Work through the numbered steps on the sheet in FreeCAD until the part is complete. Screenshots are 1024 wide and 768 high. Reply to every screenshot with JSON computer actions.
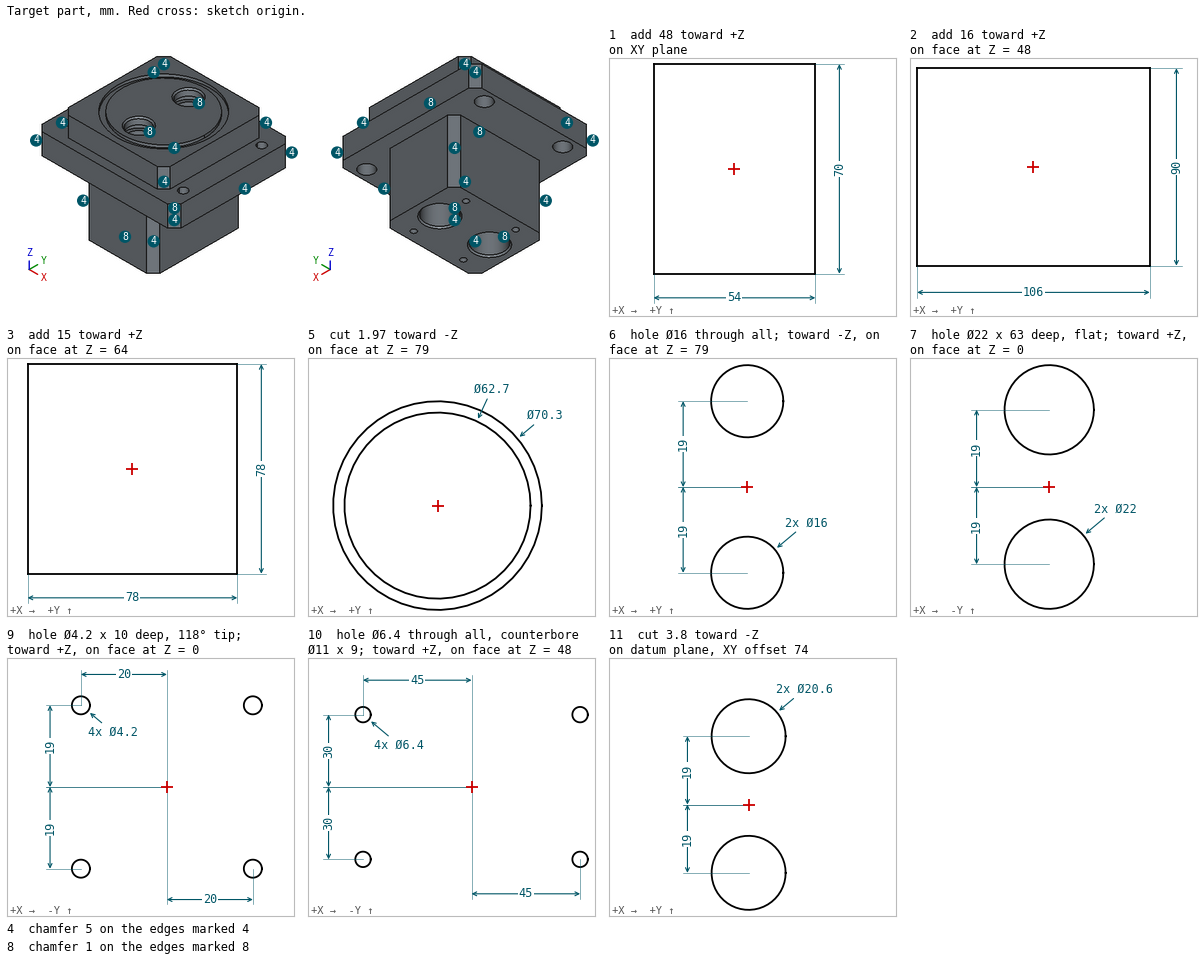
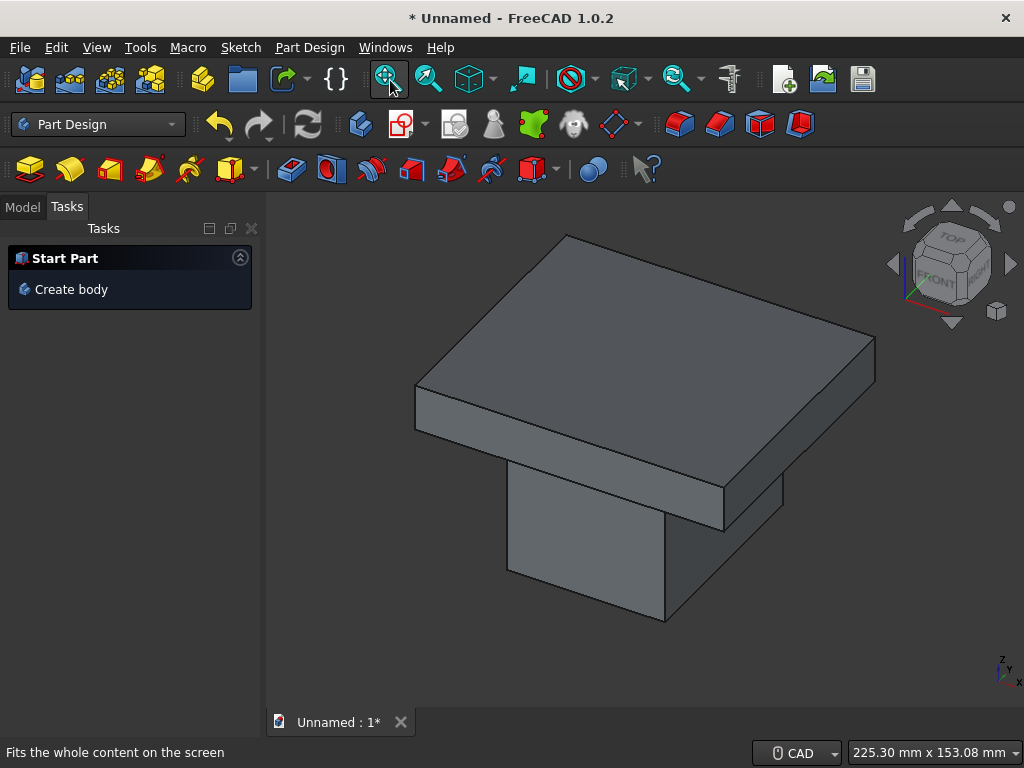
{"action": "left_click", "coordinate": [645, 360]}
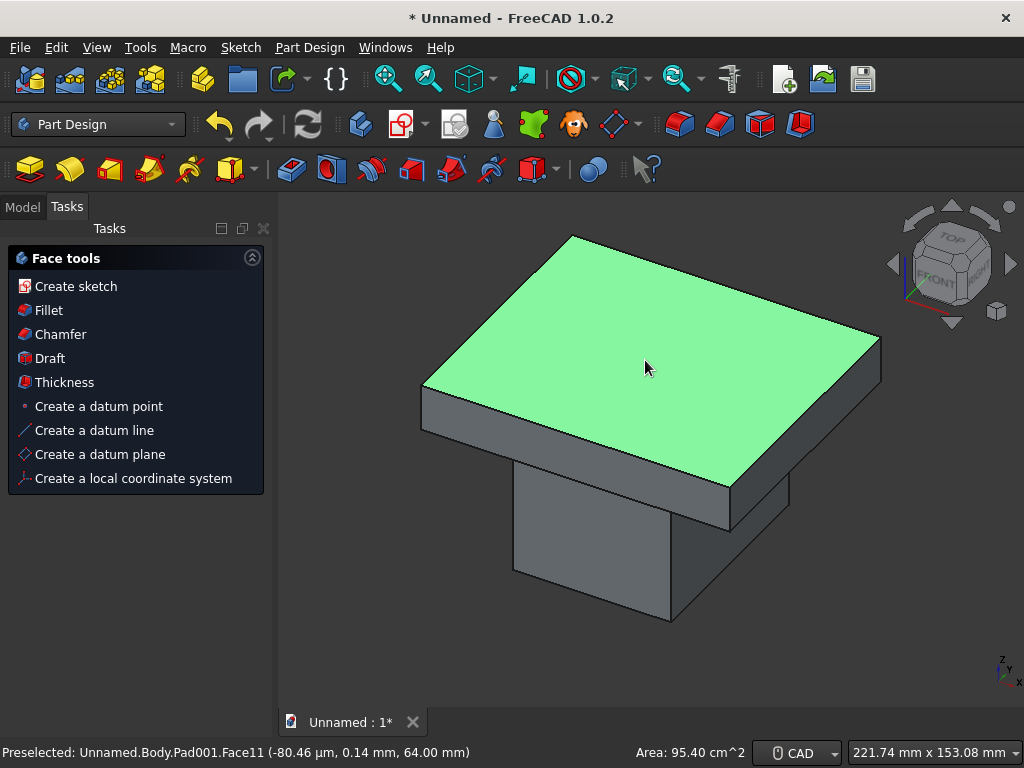
{"action": "left_click", "coordinate": [402, 124]}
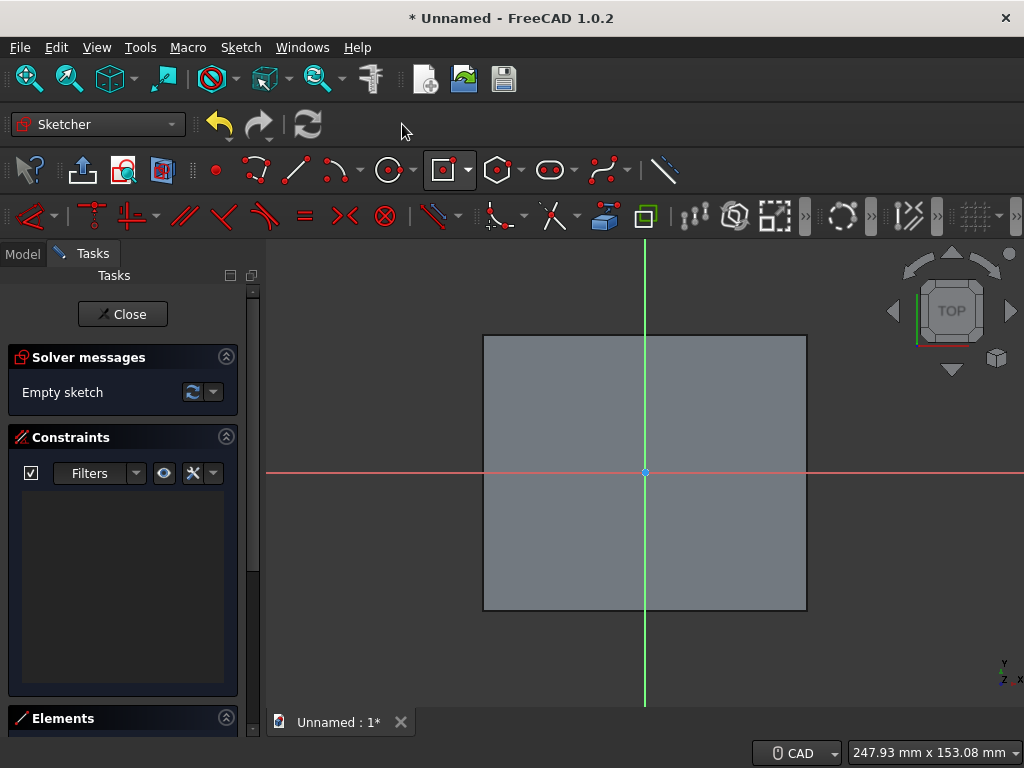
{"action": "left_click", "coordinate": [444, 170]}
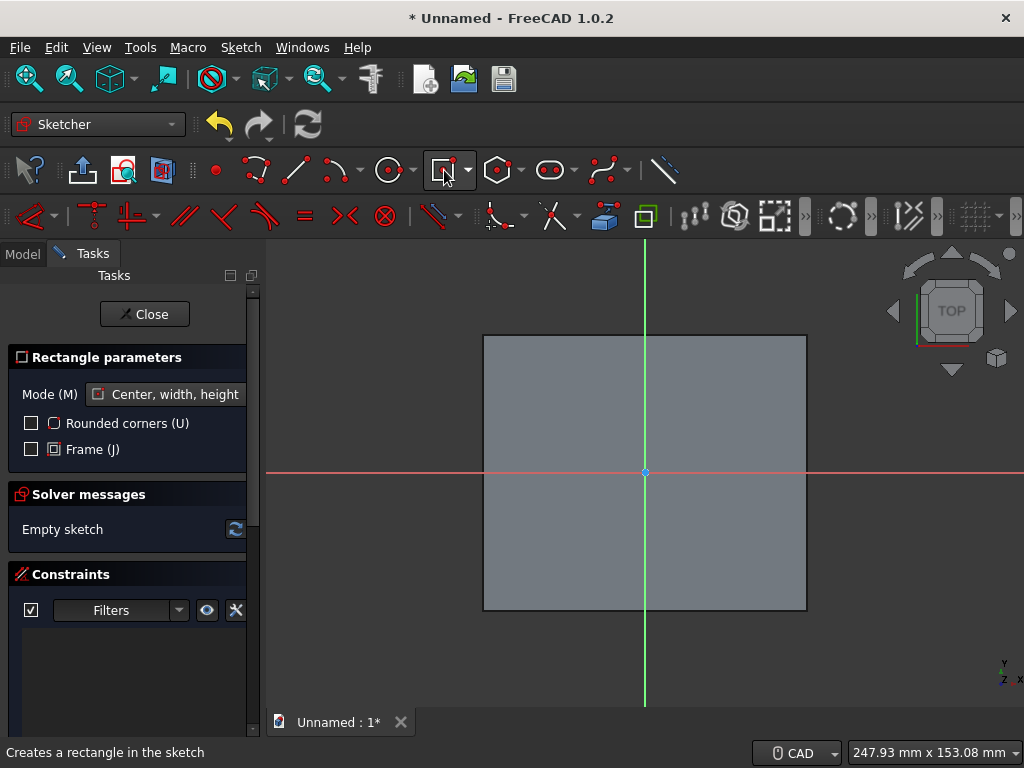
{"action": "left_click", "coordinate": [645, 473]}
{"action": "mouse_move", "coordinate": [764, 354]}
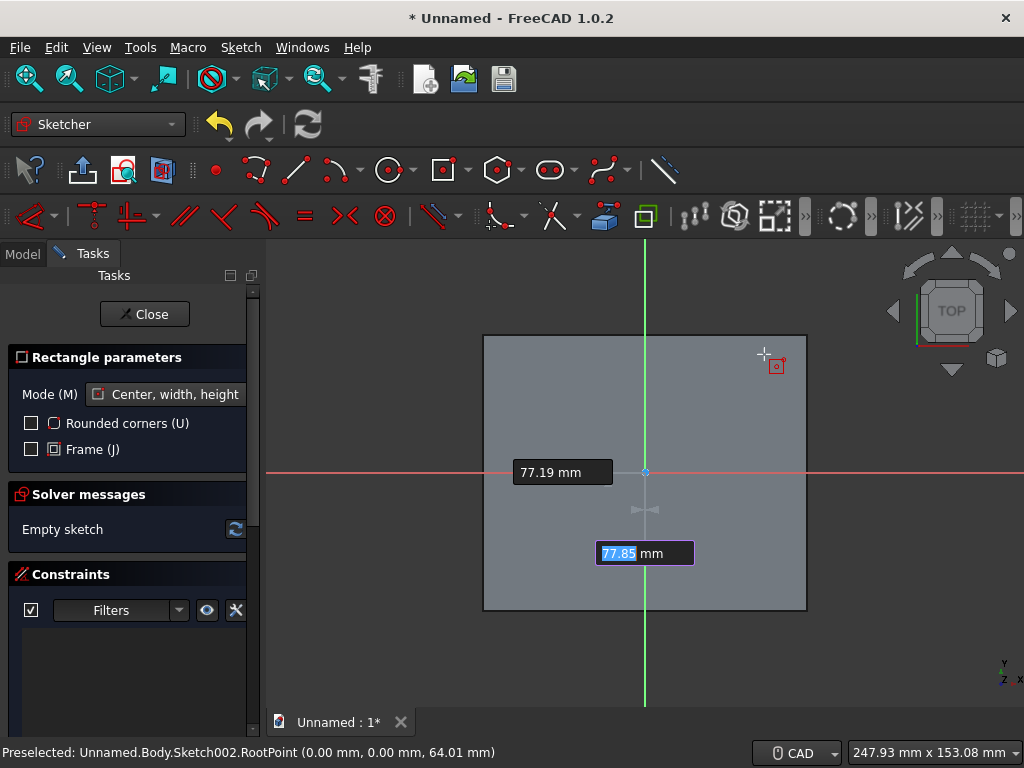
{"action": "type", "text": "78"}
{"action": "key", "text": "Tab"}
{"action": "type", "text": "78"}
{"action": "key", "text": "Return"}
{"action": "key", "text": "Escape"}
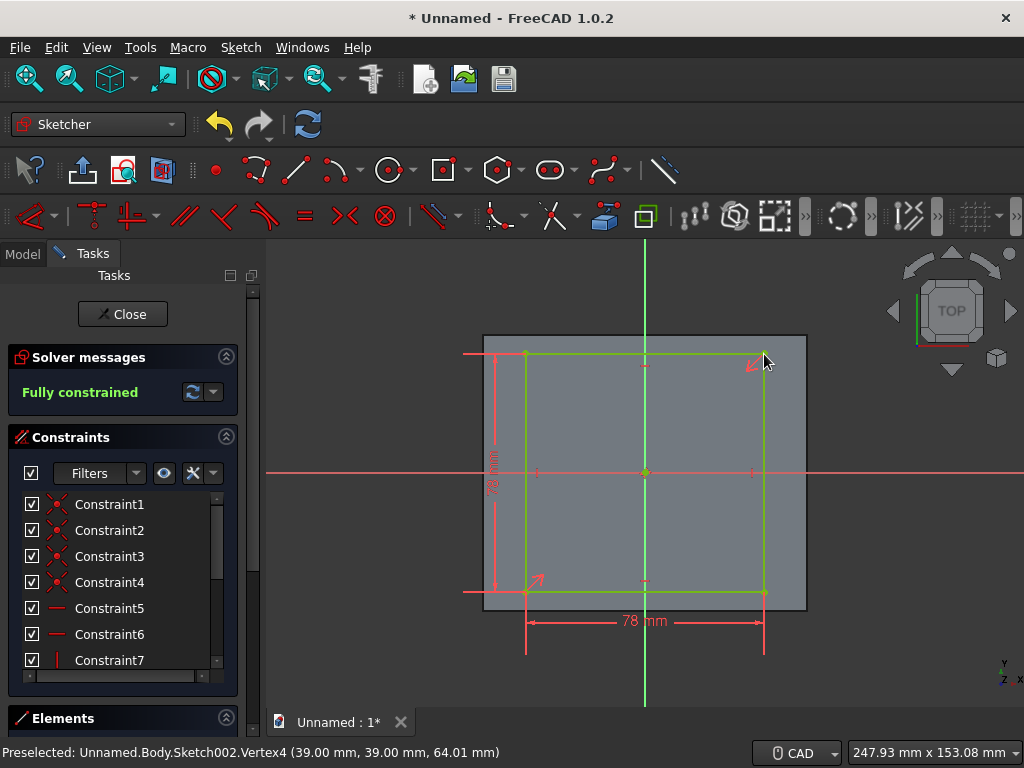
{"action": "left_click", "coordinate": [123, 314]}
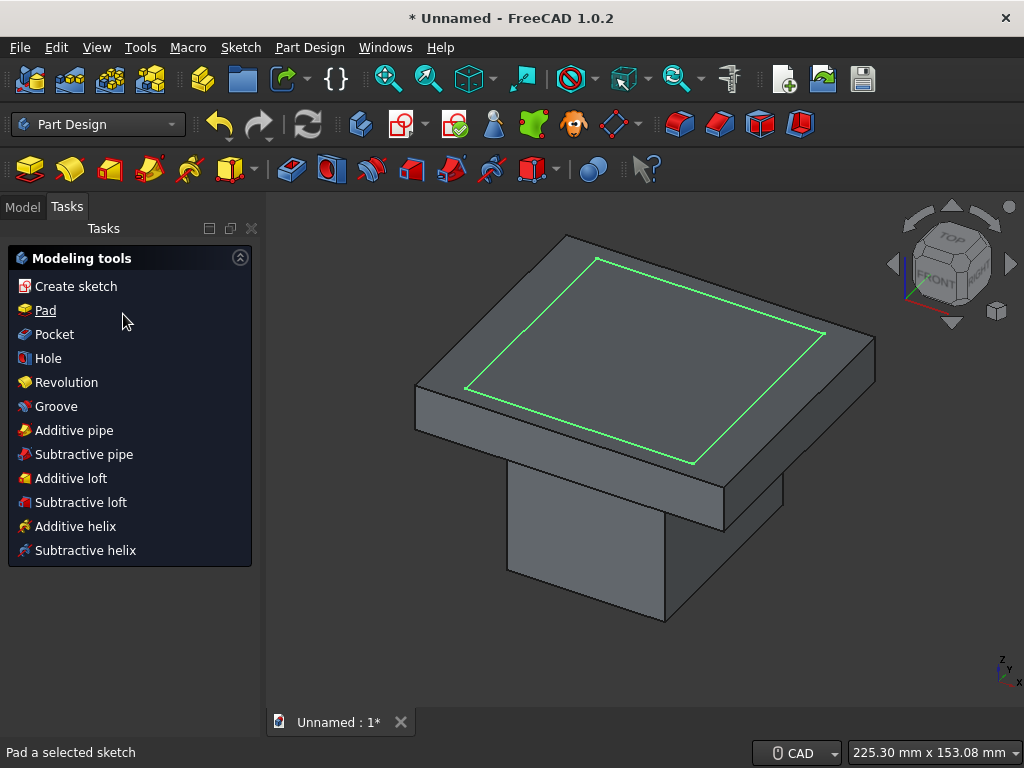
{"action": "left_click", "coordinate": [30, 170]}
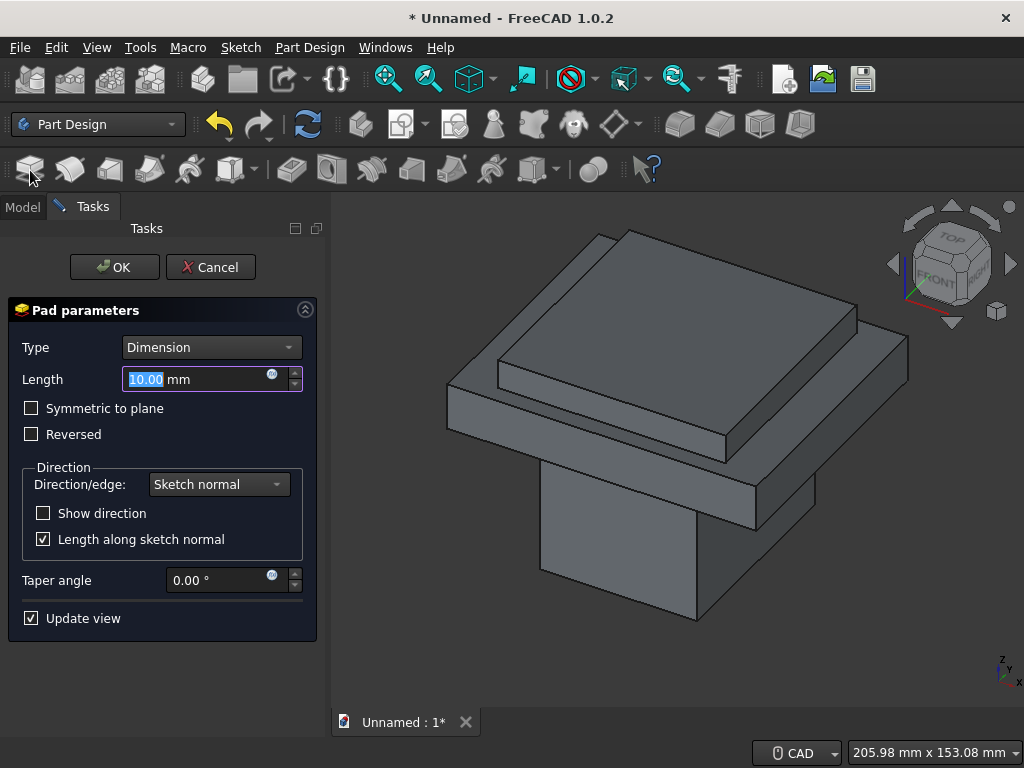
{"action": "type", "text": "15"}
{"action": "key", "text": "Tab"}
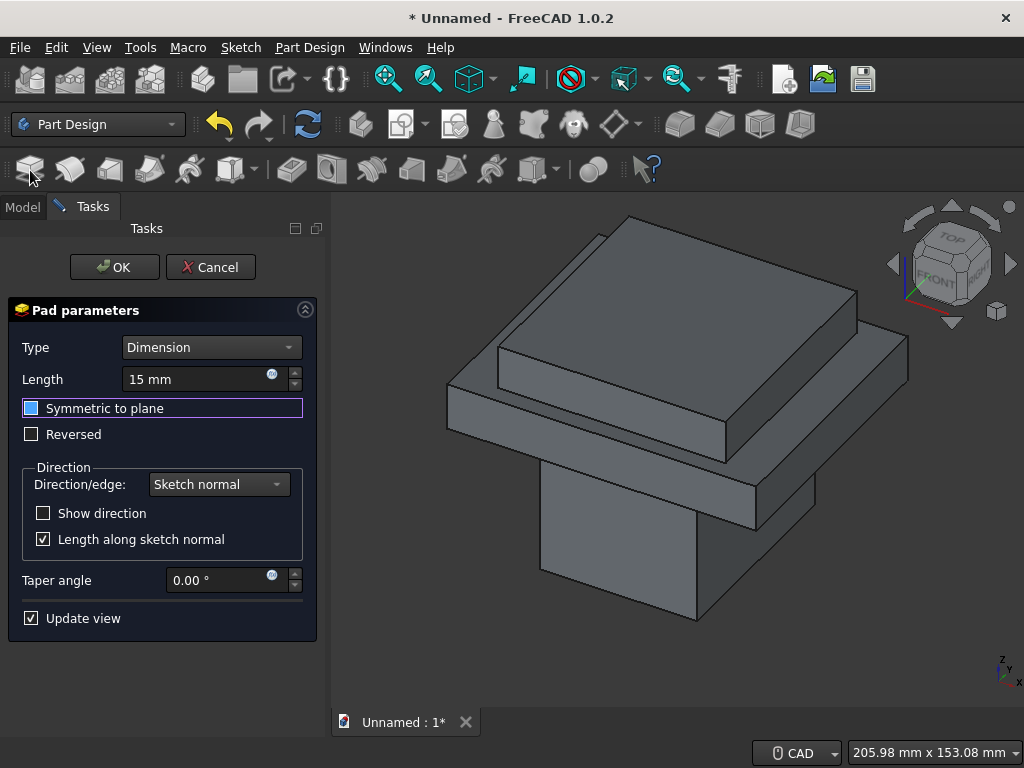
{"action": "left_click", "coordinate": [115, 267]}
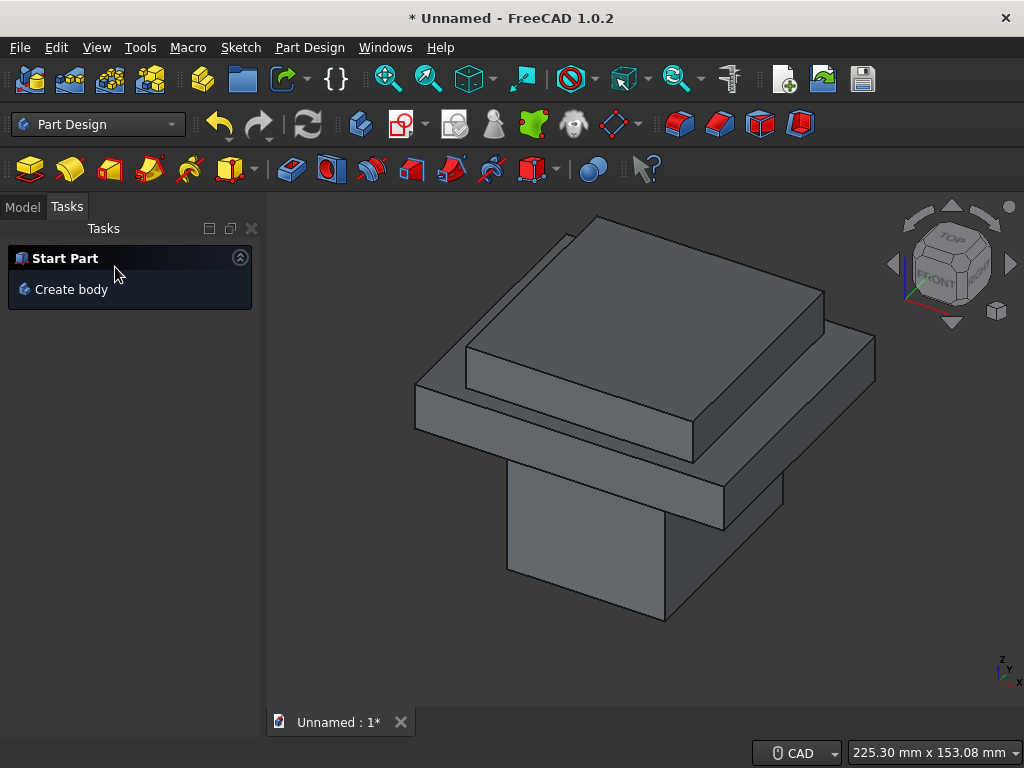
{"action": "left_click", "coordinate": [724, 508]}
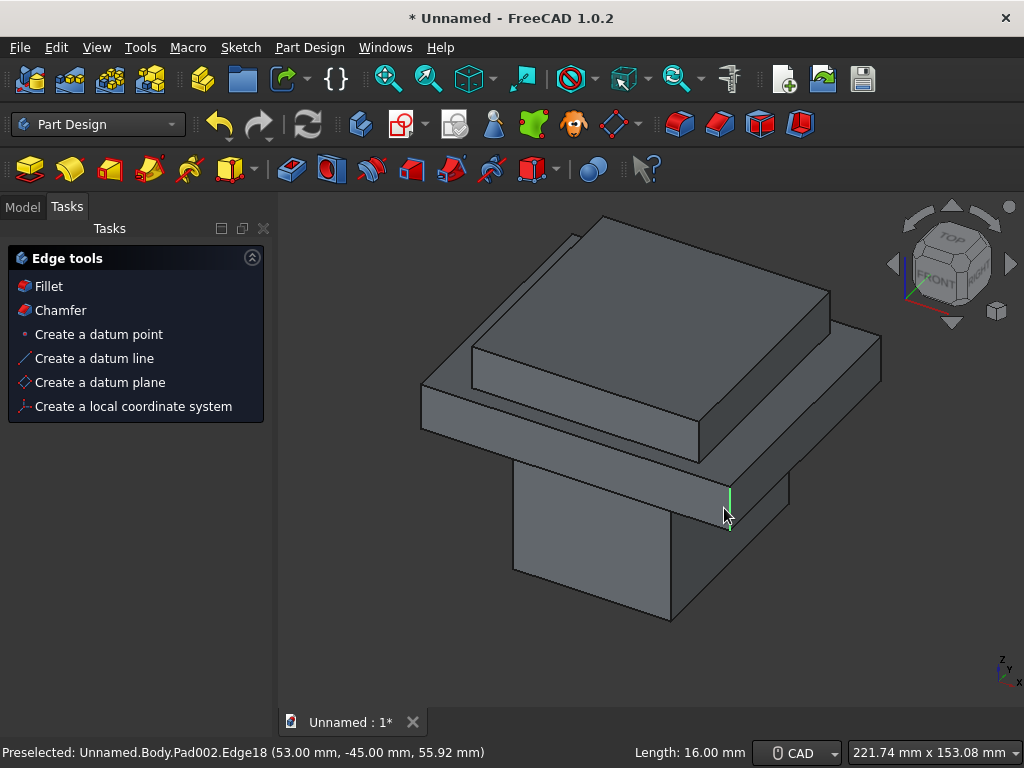
{"action": "left_click", "coordinate": [699, 442], "text": "ctrl"}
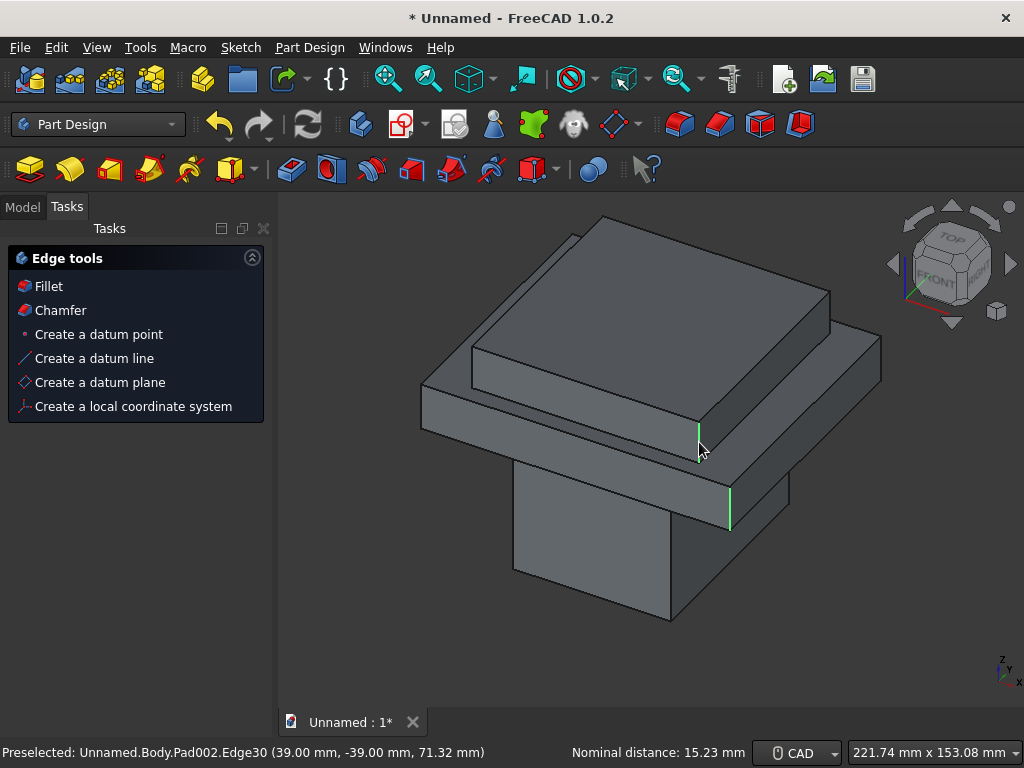
{"action": "left_click", "coordinate": [671, 554], "text": "ctrl"}